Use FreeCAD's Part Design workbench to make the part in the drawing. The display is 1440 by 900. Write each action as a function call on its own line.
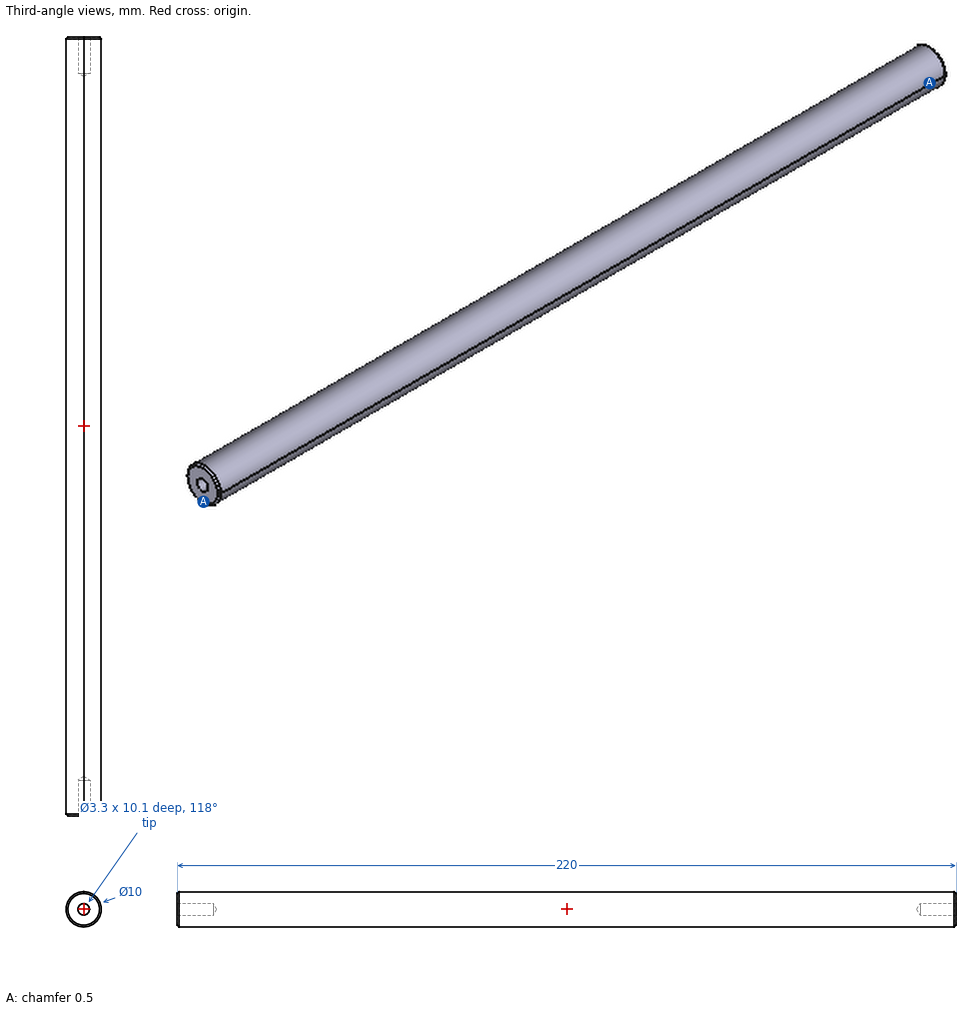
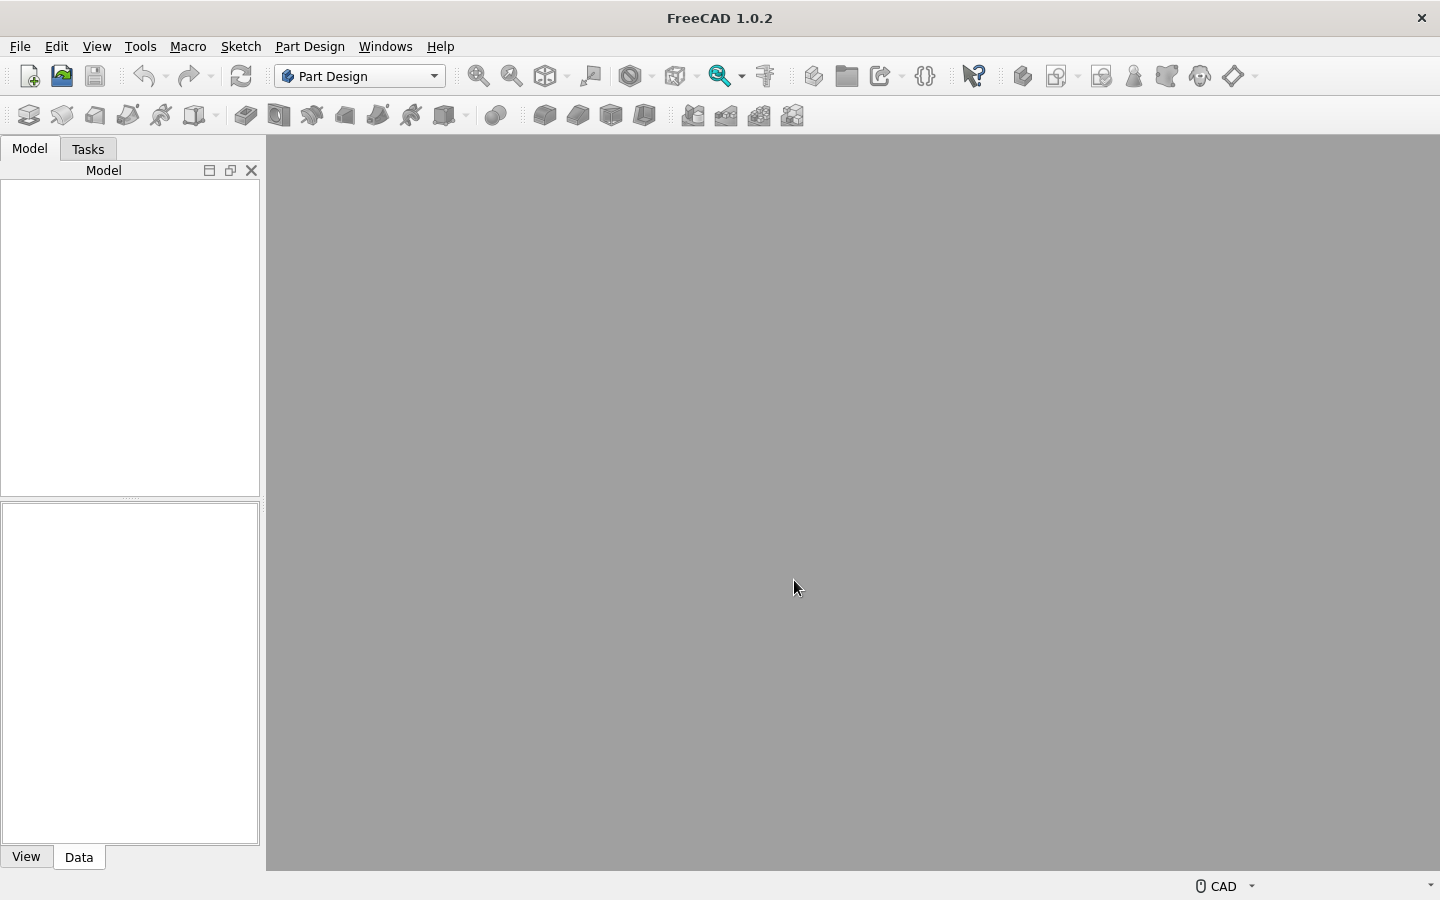
key(ctrl+n)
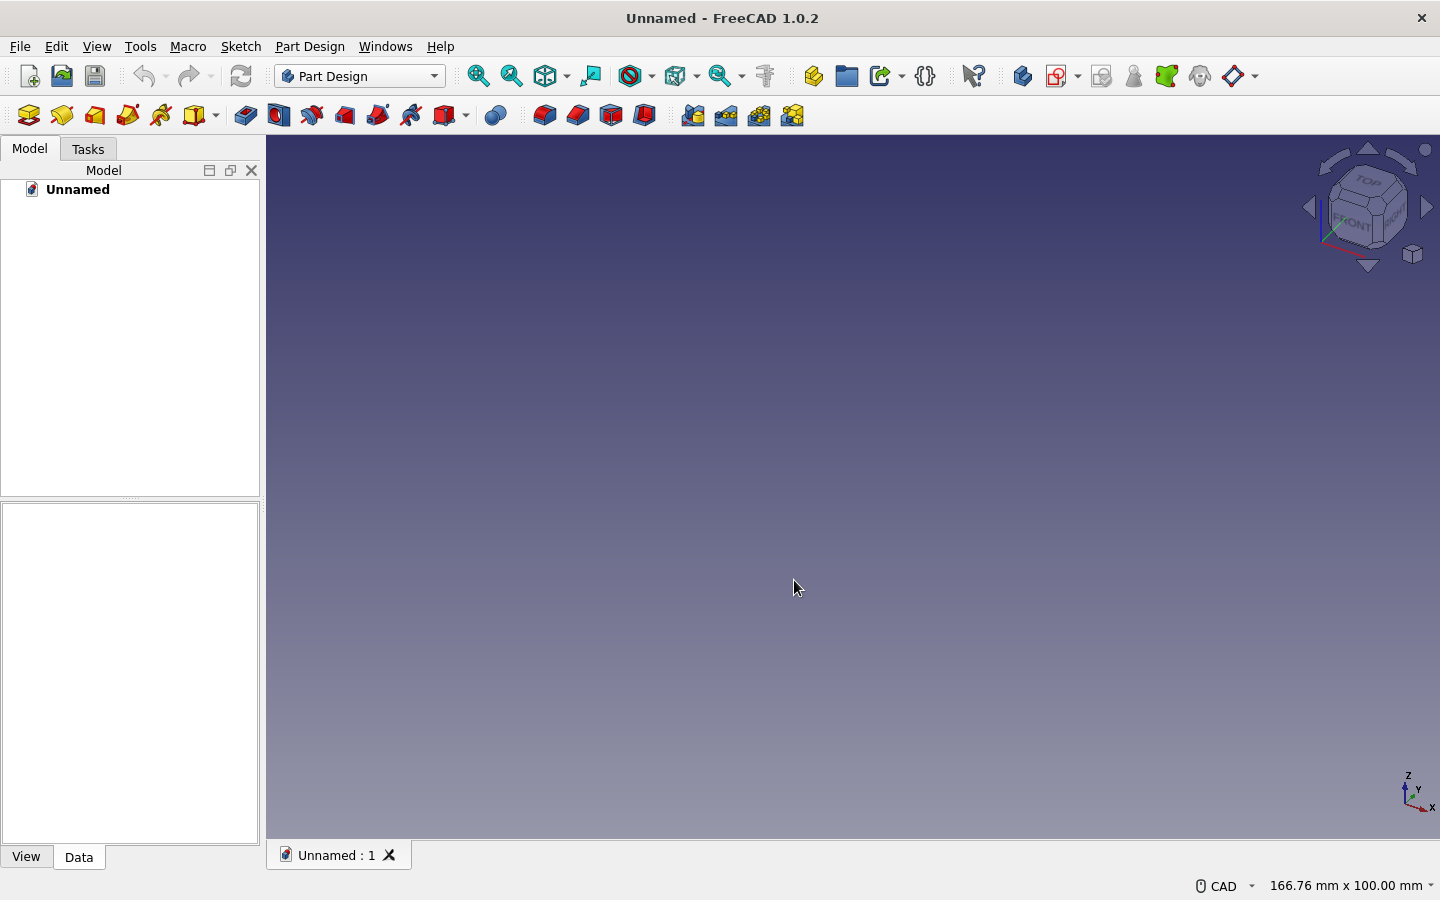
click(1056, 76)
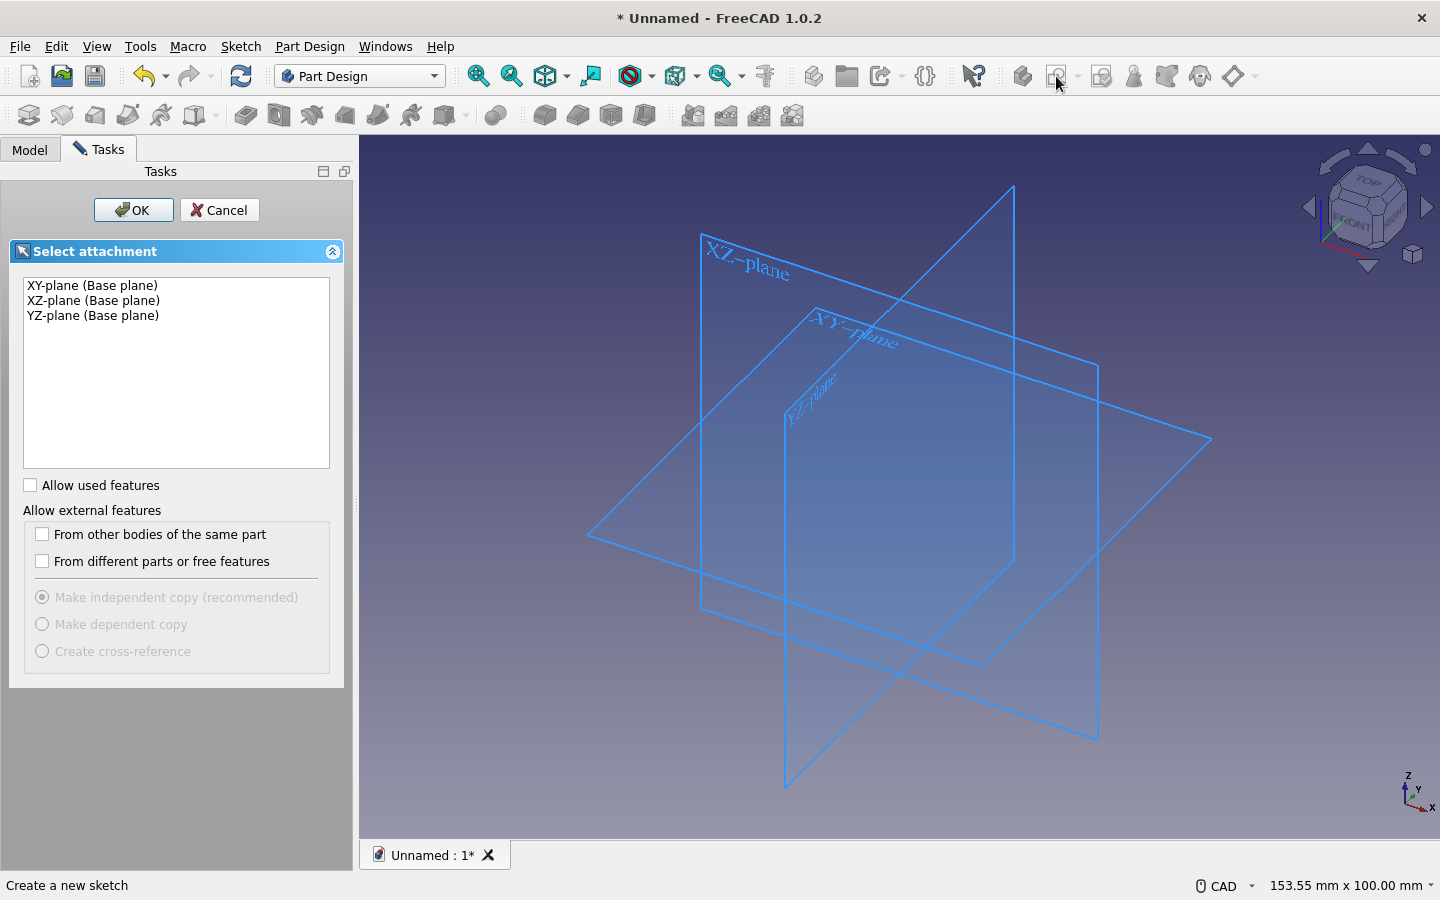
click(84, 300)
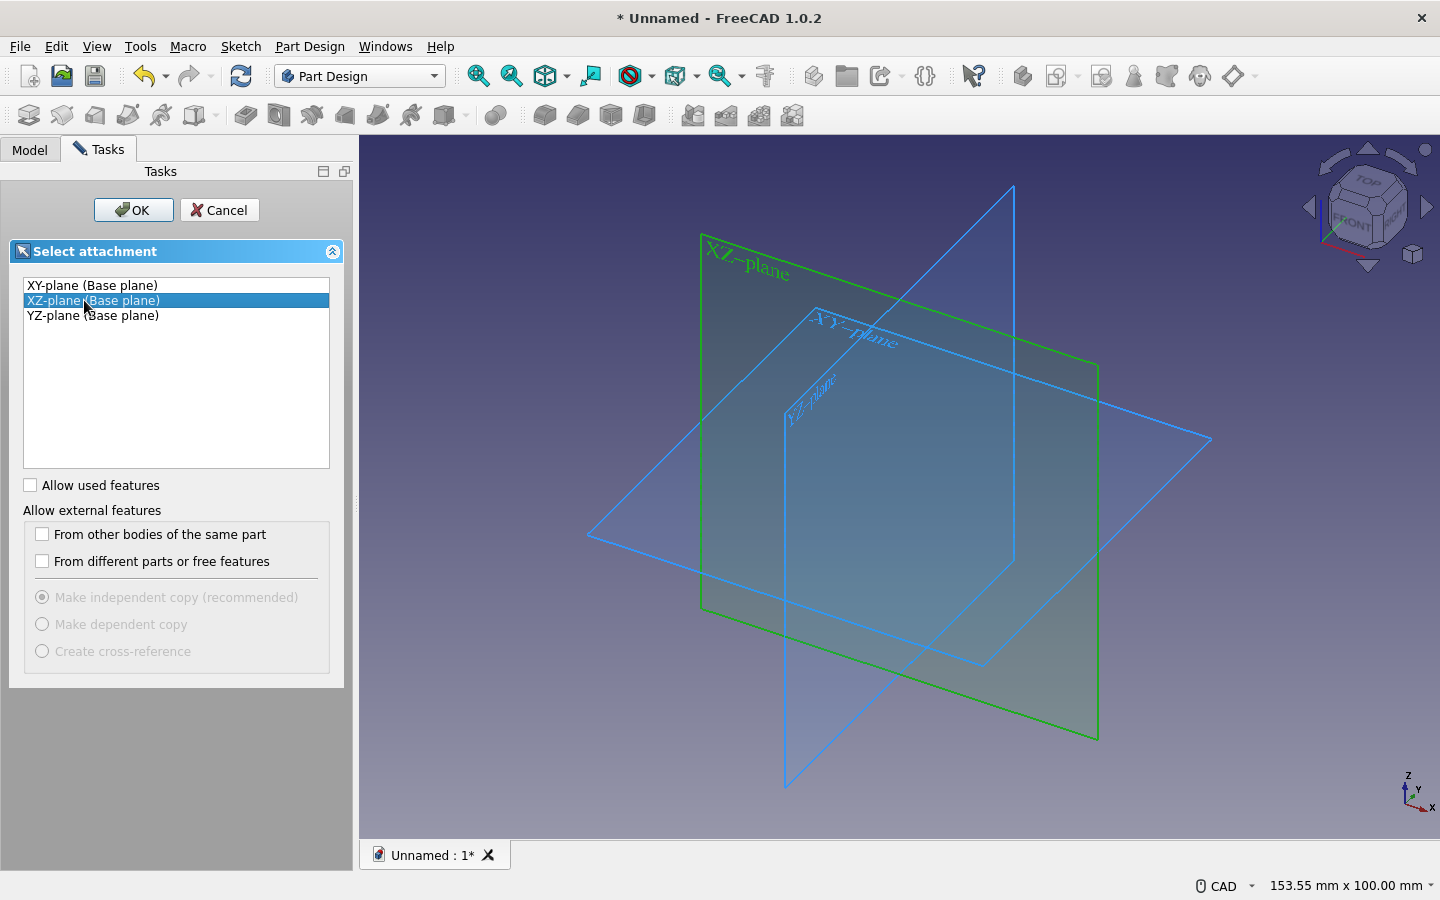
click(134, 210)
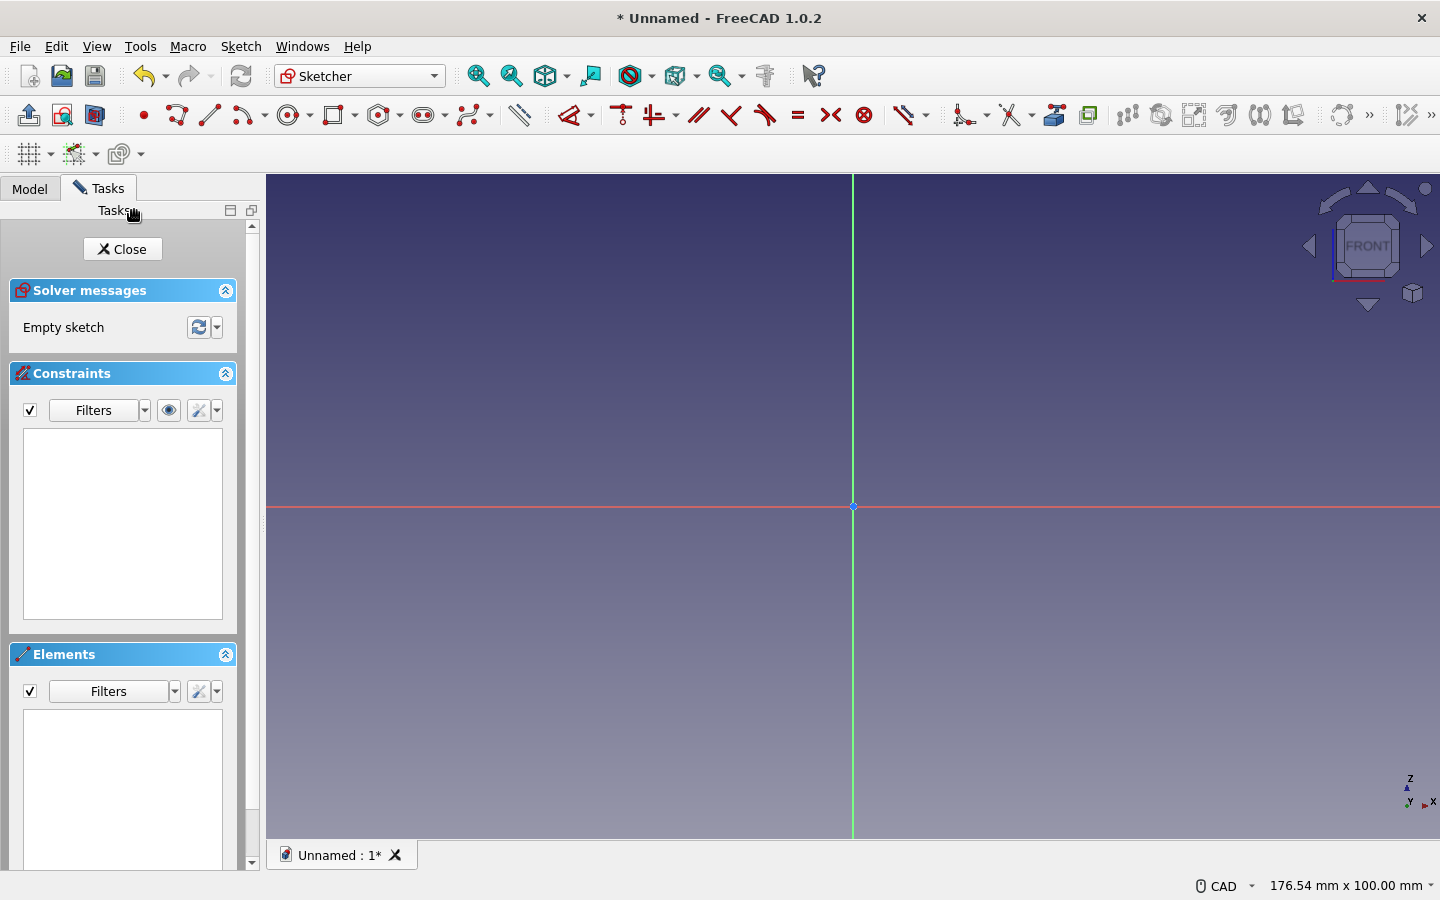
scroll(867, 506, up, 9)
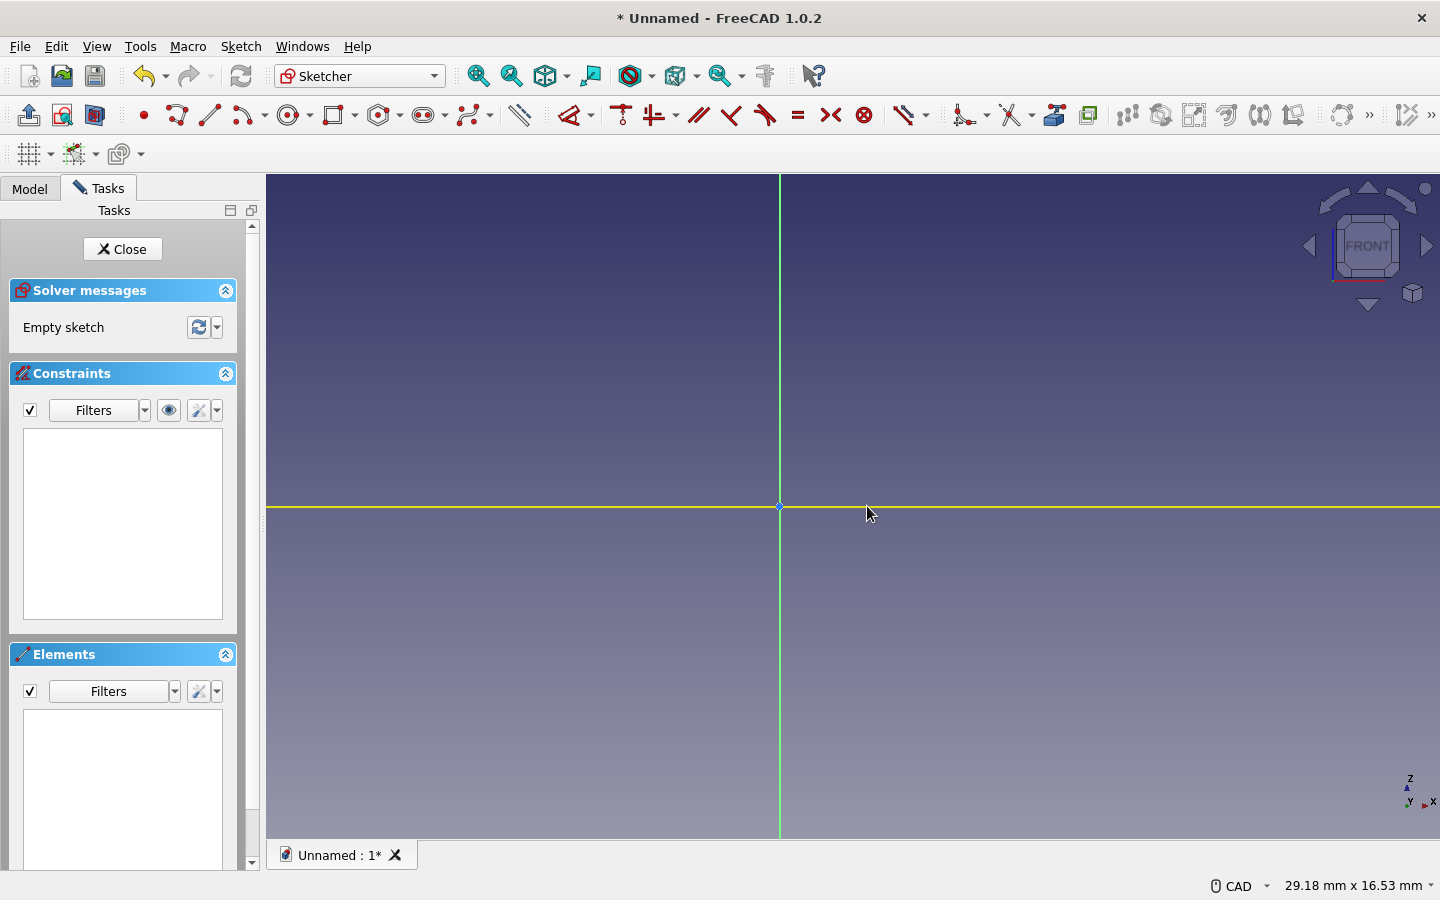
key(g)
key(c)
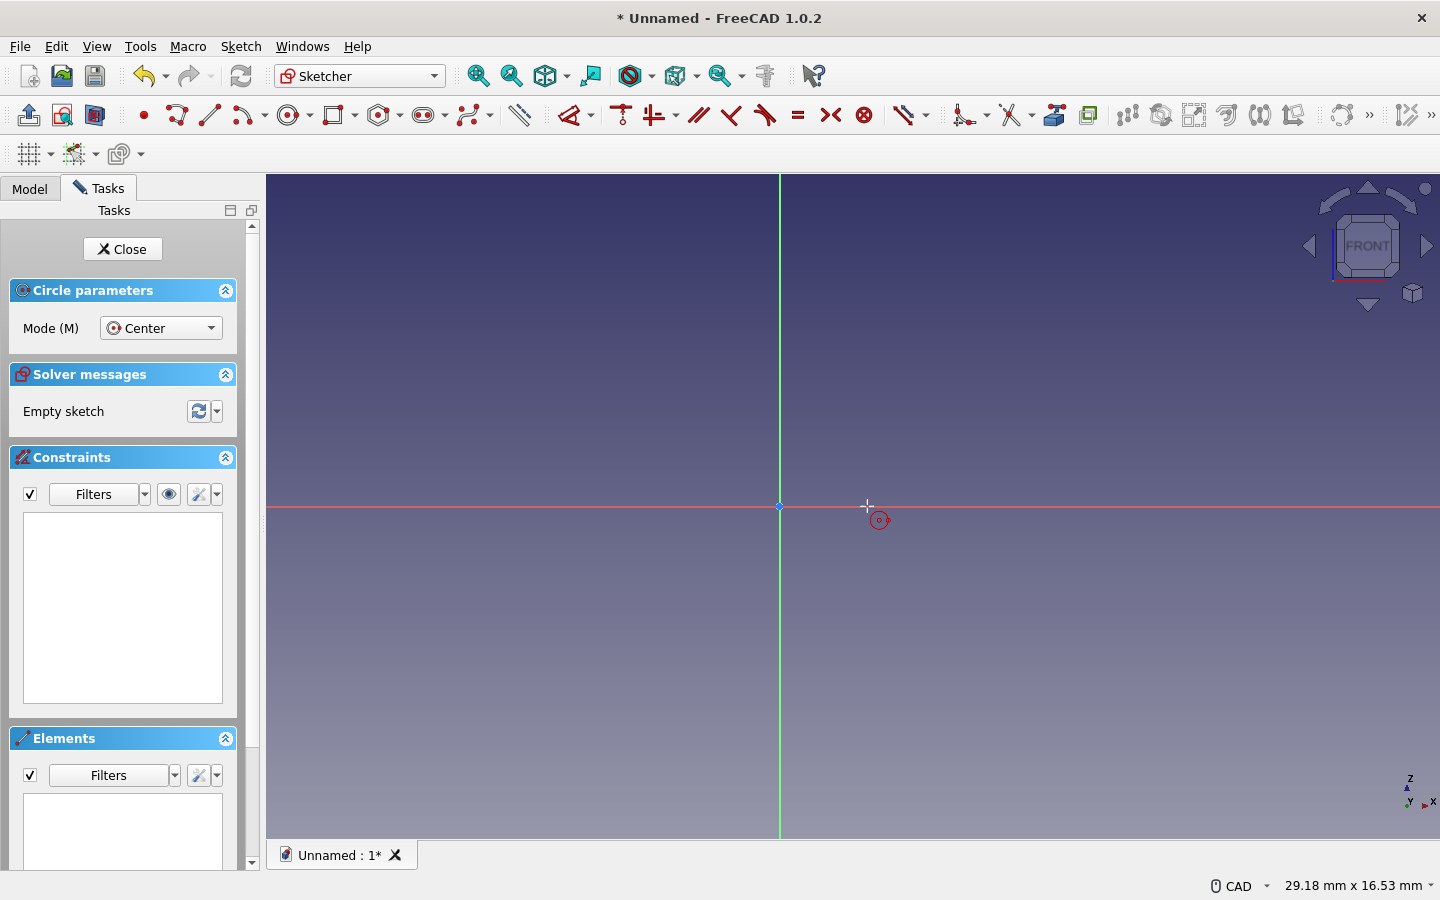
click(780, 506)
move(922, 364)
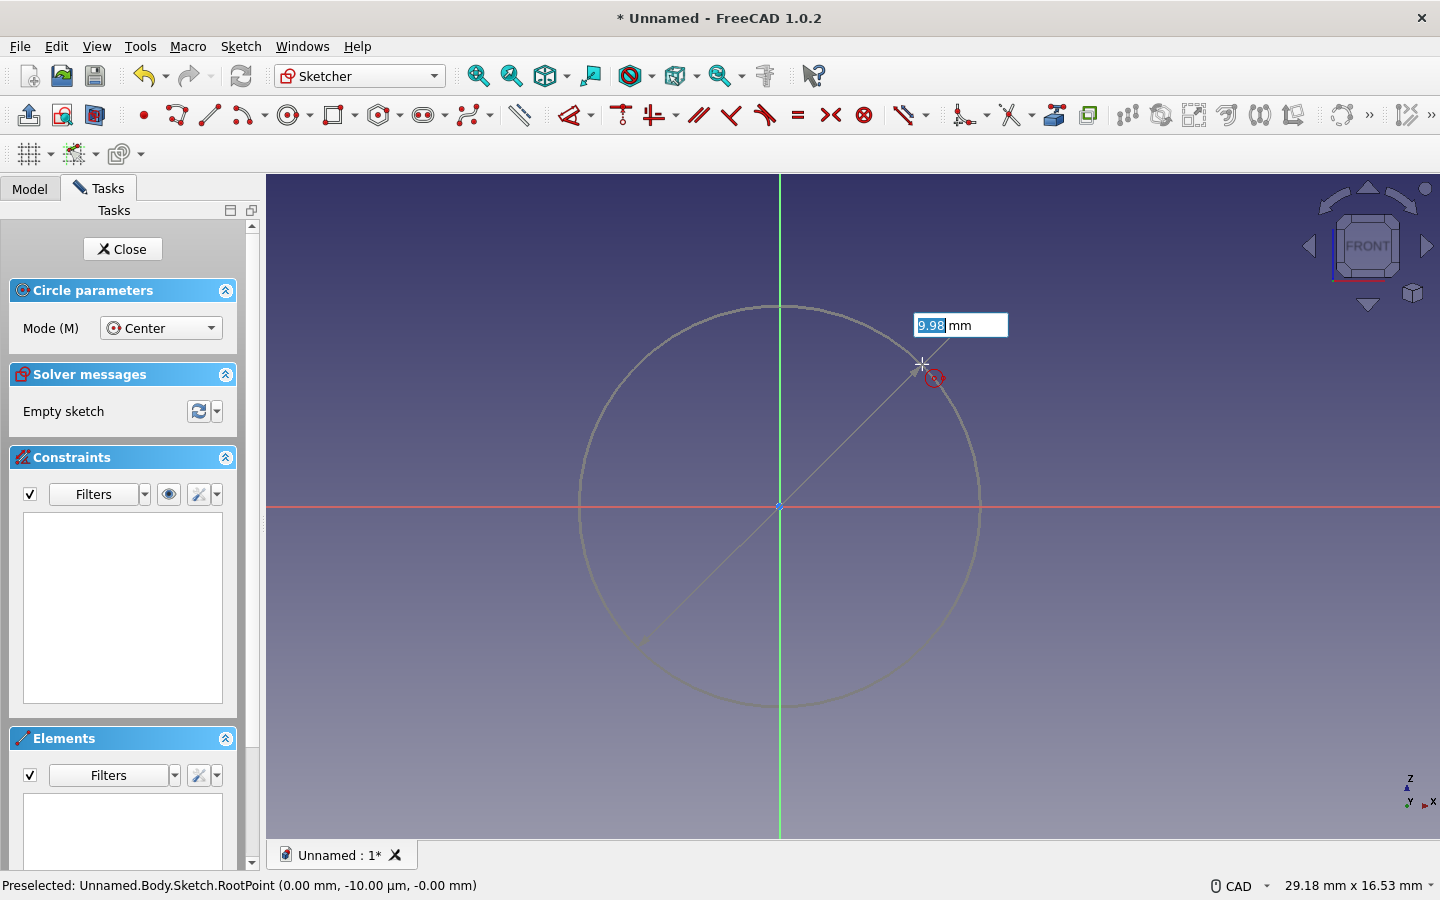
text(10)
key(Return)
key(Escape)